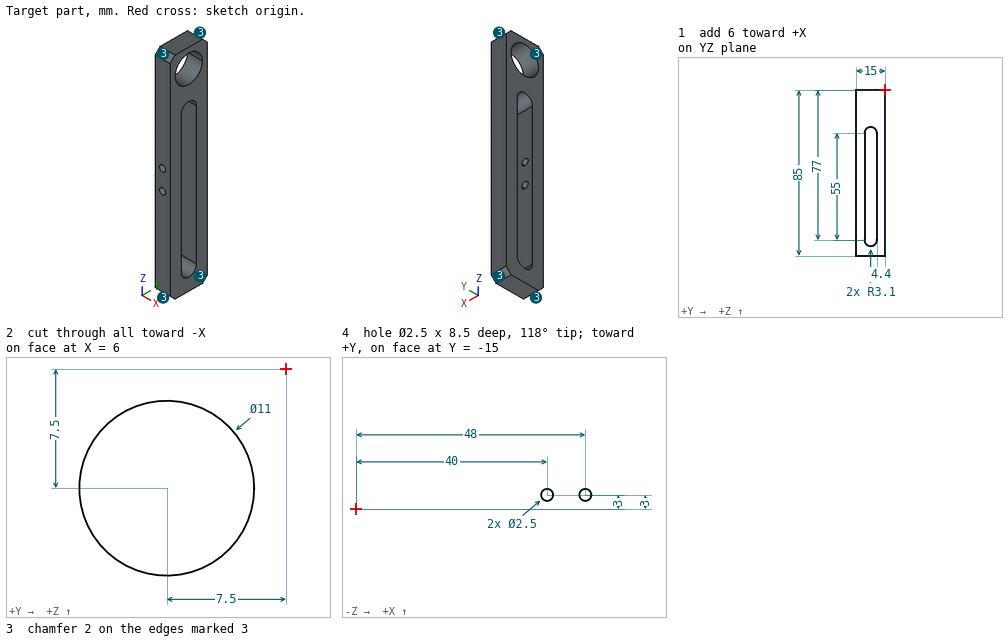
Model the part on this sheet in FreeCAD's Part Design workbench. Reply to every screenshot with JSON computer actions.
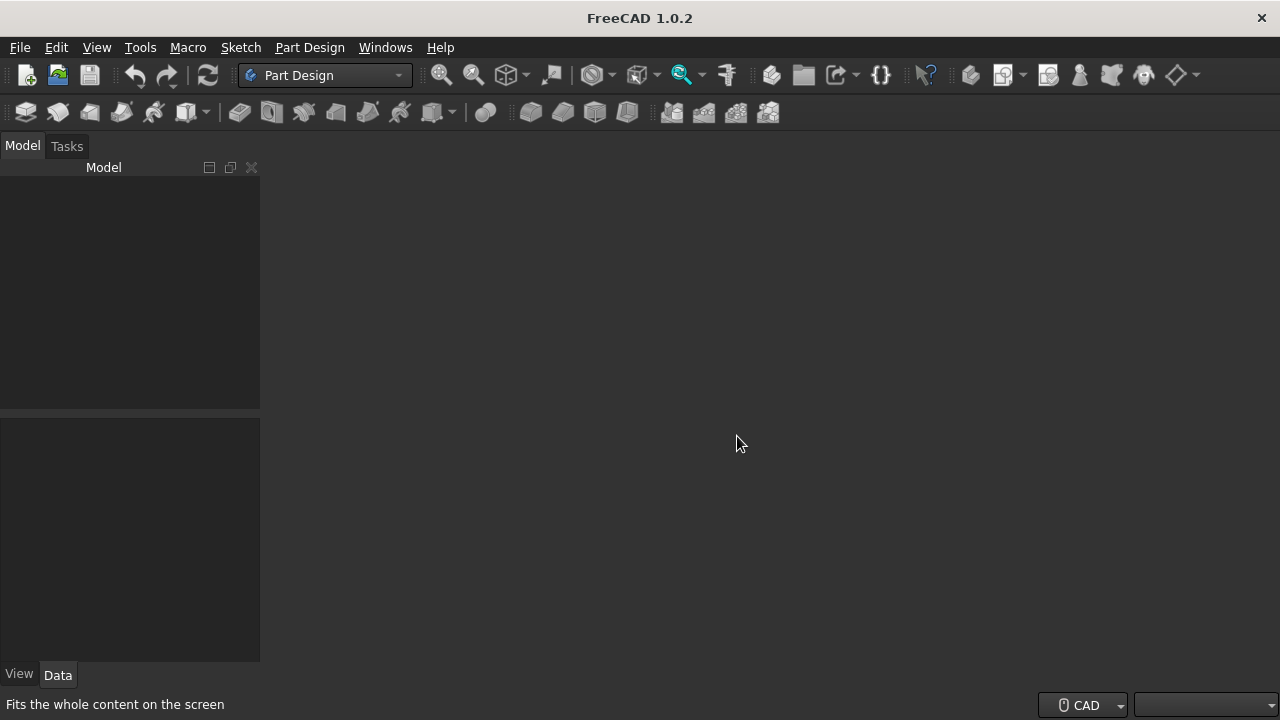
{"action": "key", "text": "ctrl+n"}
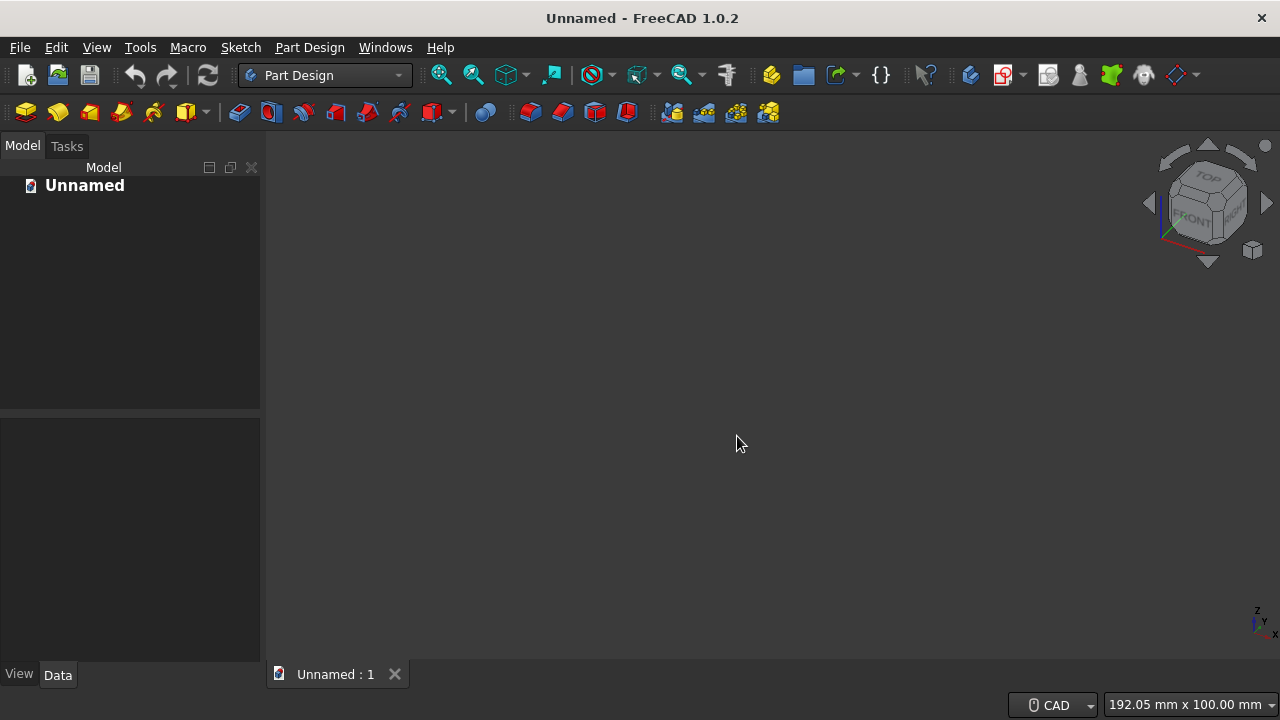
{"action": "left_click", "coordinate": [1004, 76]}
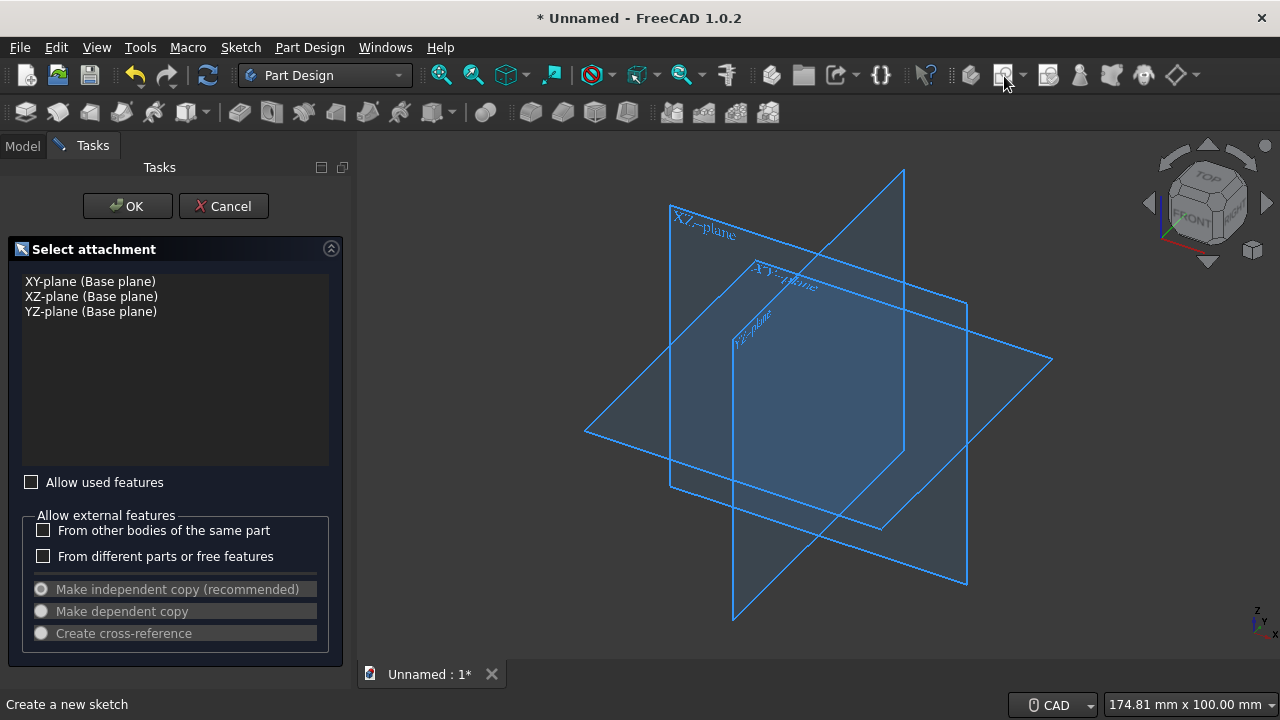
{"action": "left_click", "coordinate": [82, 312]}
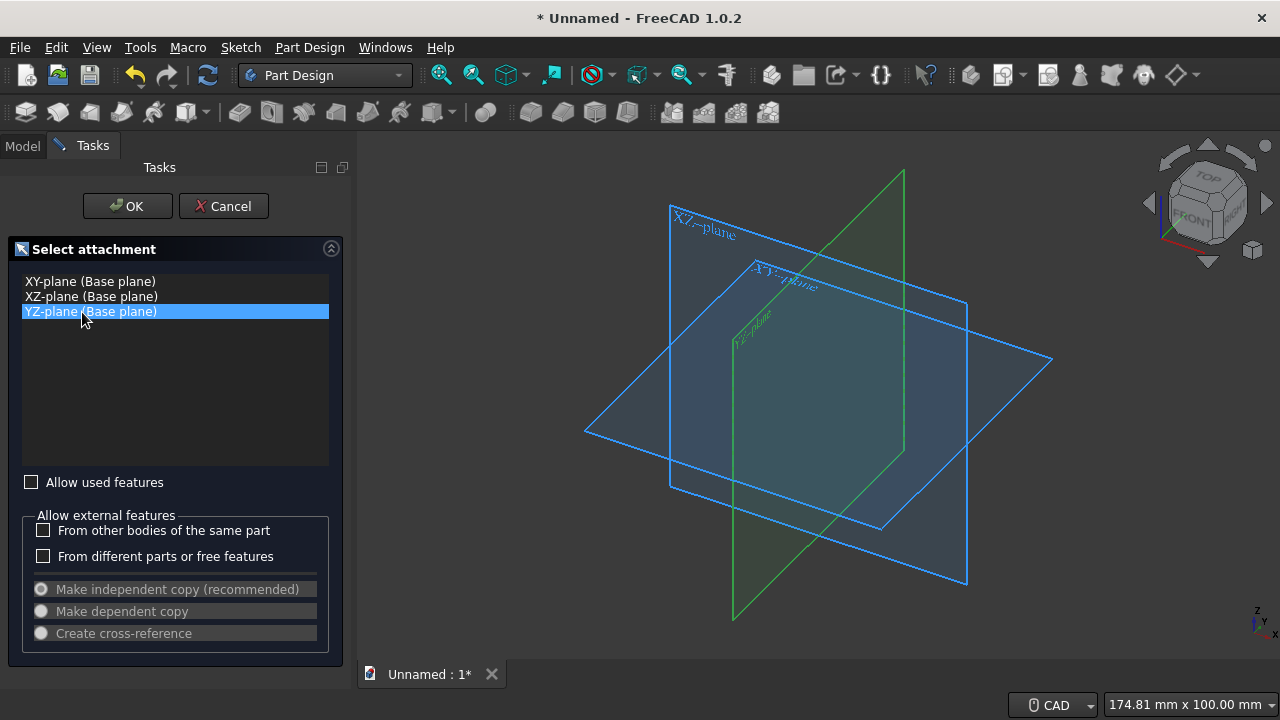
{"action": "left_click", "coordinate": [128, 206]}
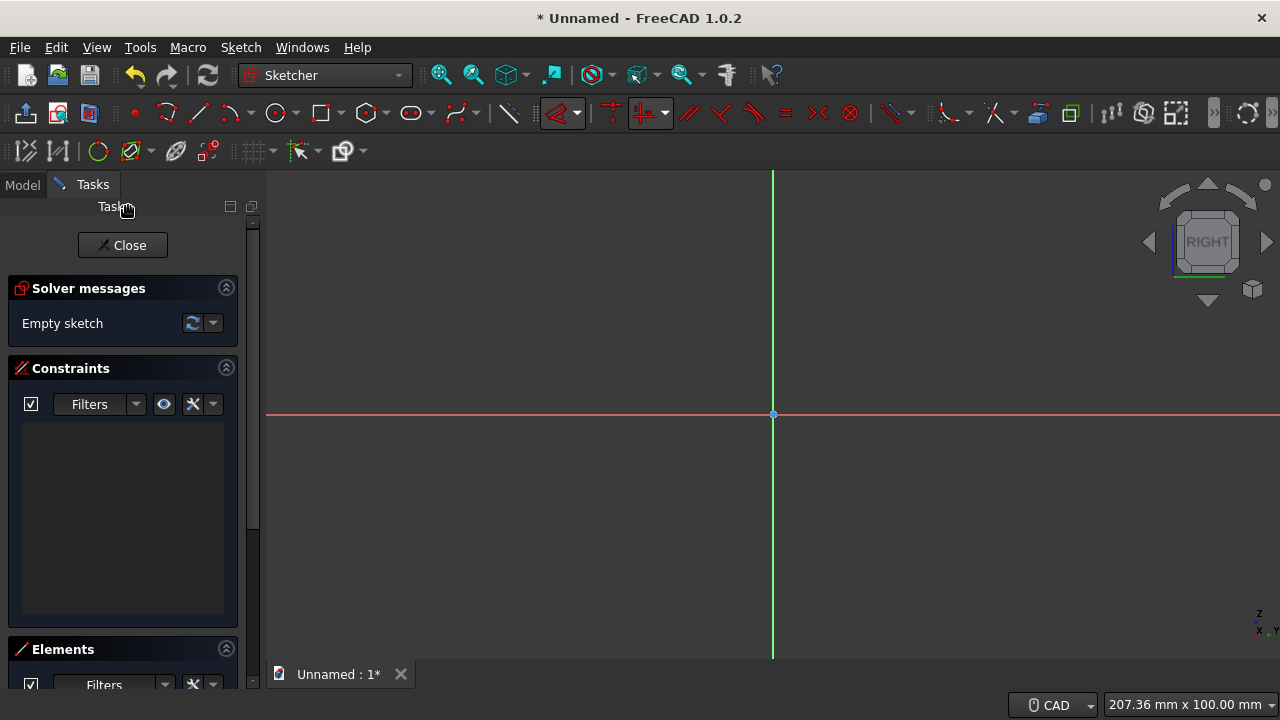
{"action": "scroll", "coordinate": [666, 198], "scroll_direction": "down", "scroll_amount": 3}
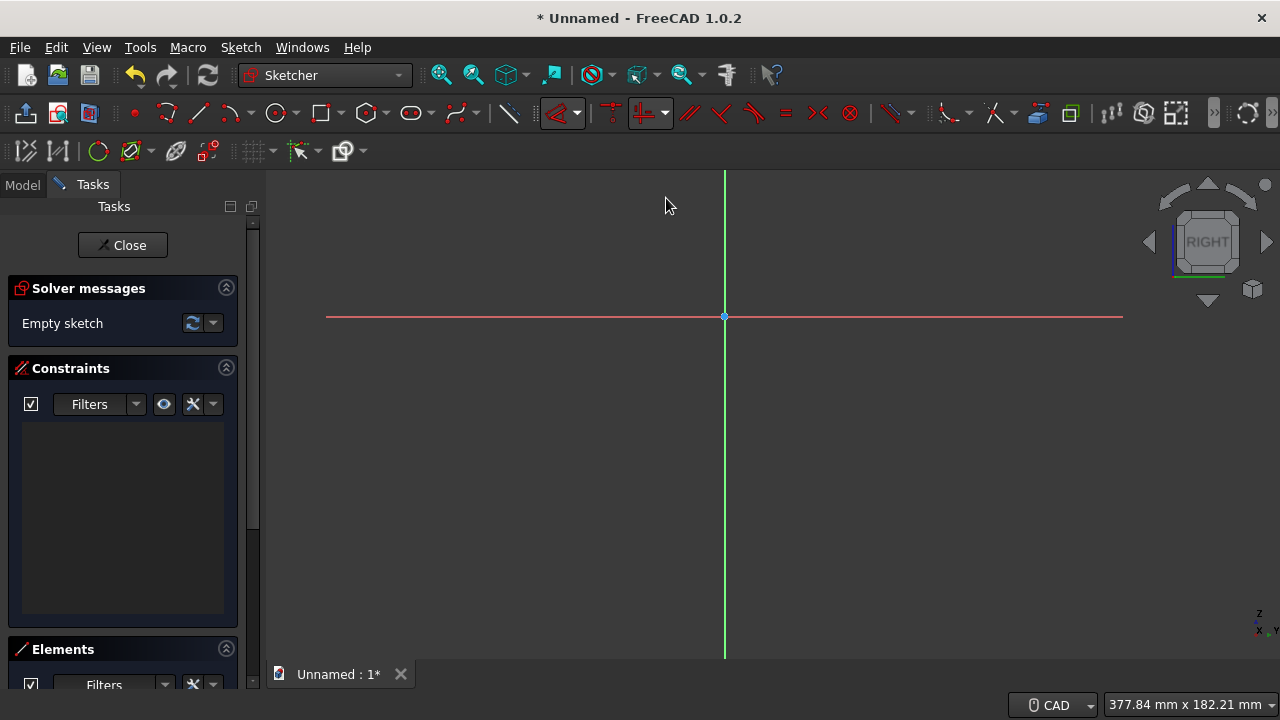
{"action": "key", "text": "g r"}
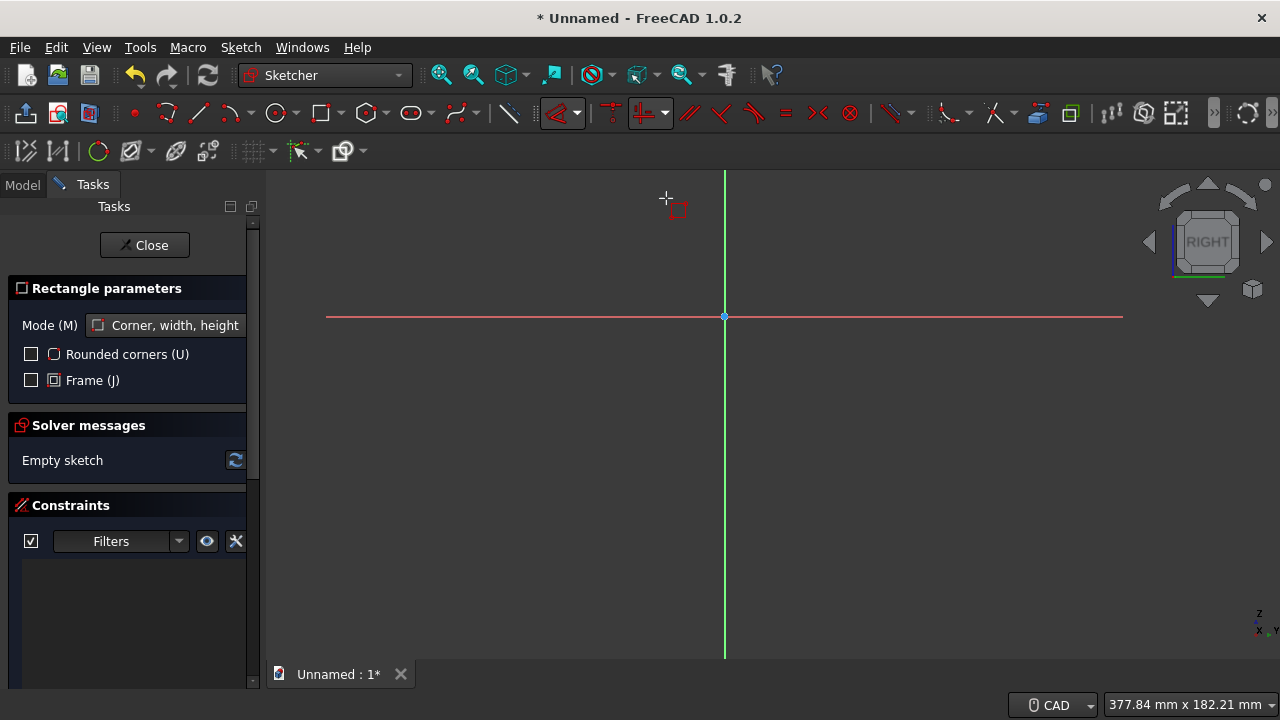
{"action": "left_click", "coordinate": [725, 317]}
{"action": "left_click", "coordinate": [685, 545]}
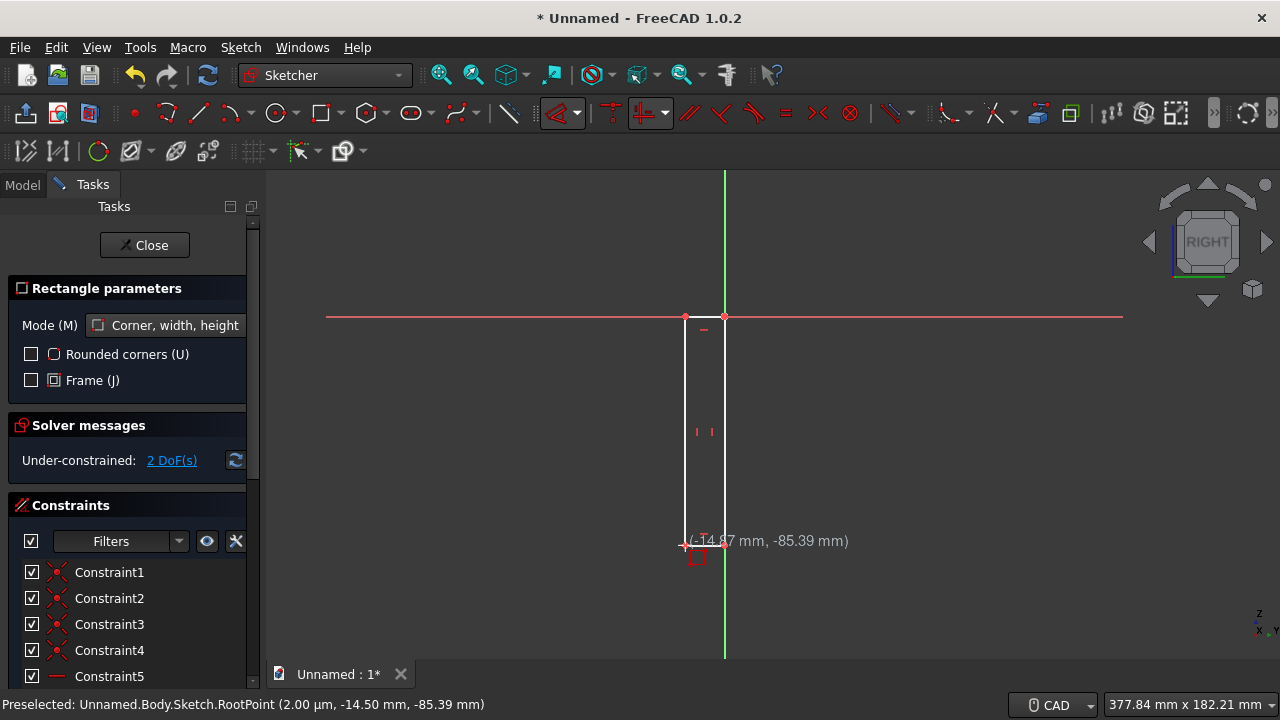
{"action": "key", "text": "g s"}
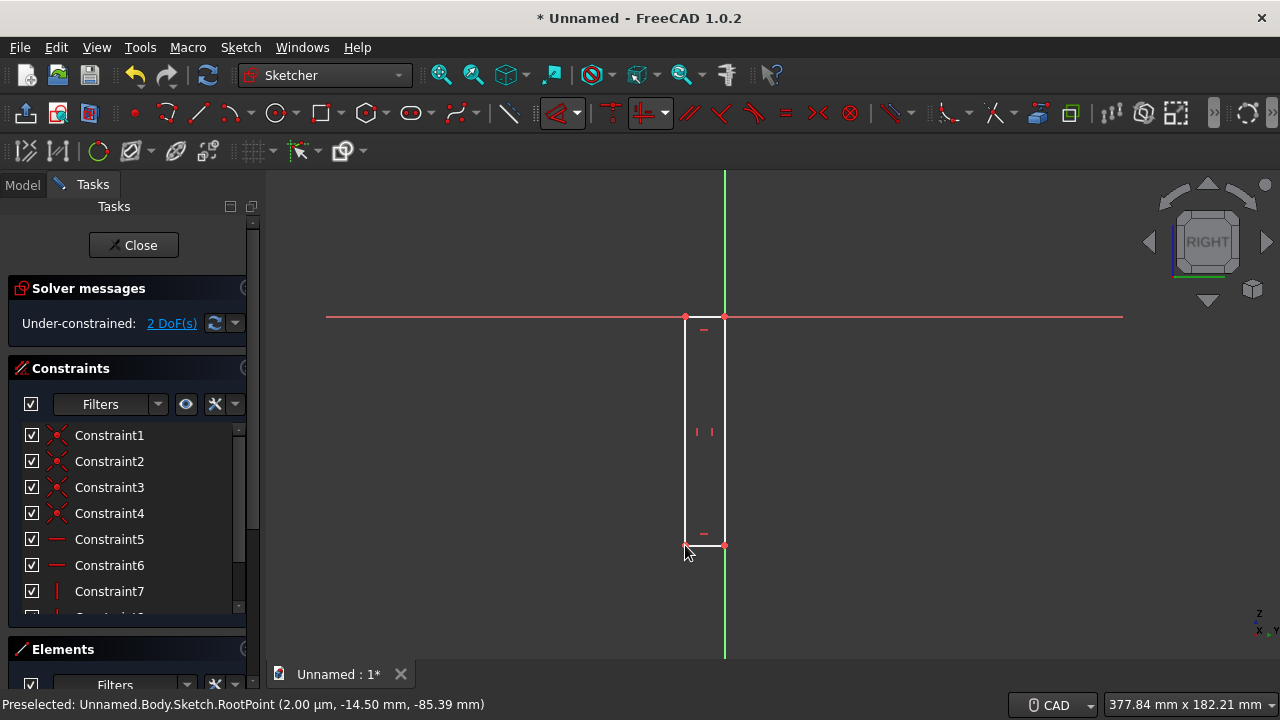
{"action": "scroll", "coordinate": [705, 523], "scroll_direction": "up", "scroll_amount": 6}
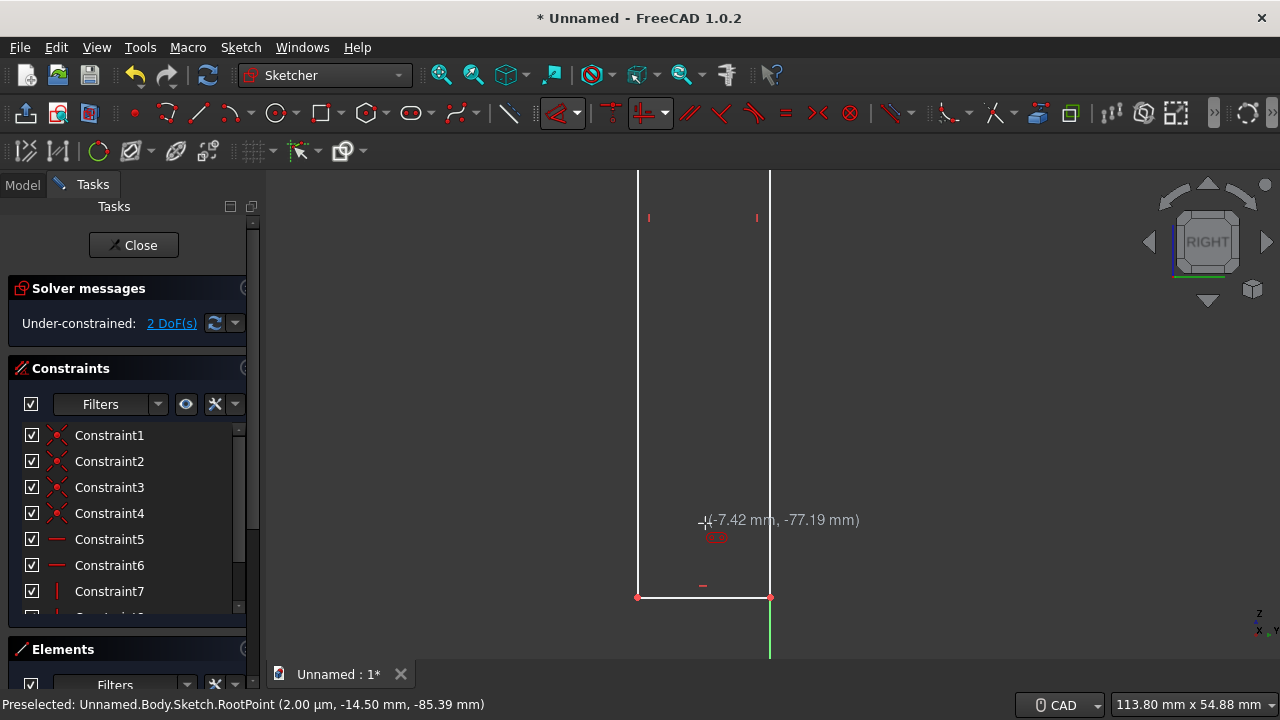
{"action": "left_click", "coordinate": [703, 523]}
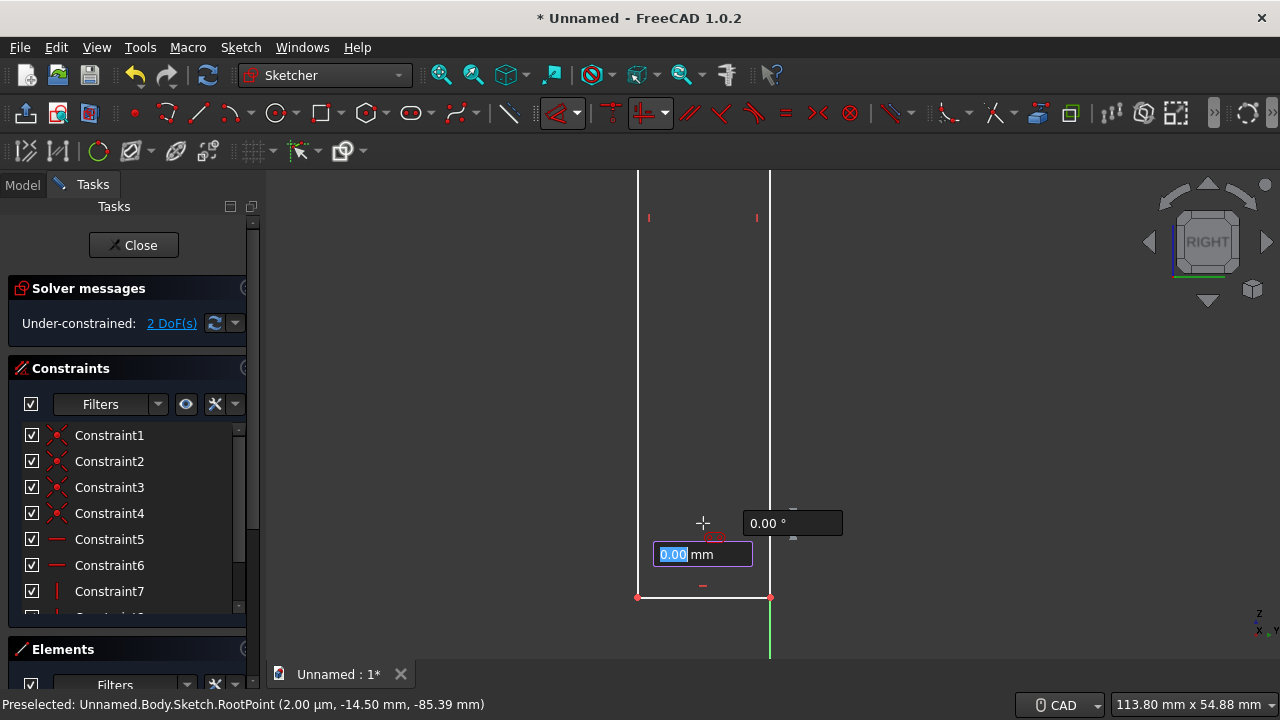
{"action": "scroll", "coordinate": [705, 530], "scroll_direction": "down", "scroll_amount": 5}